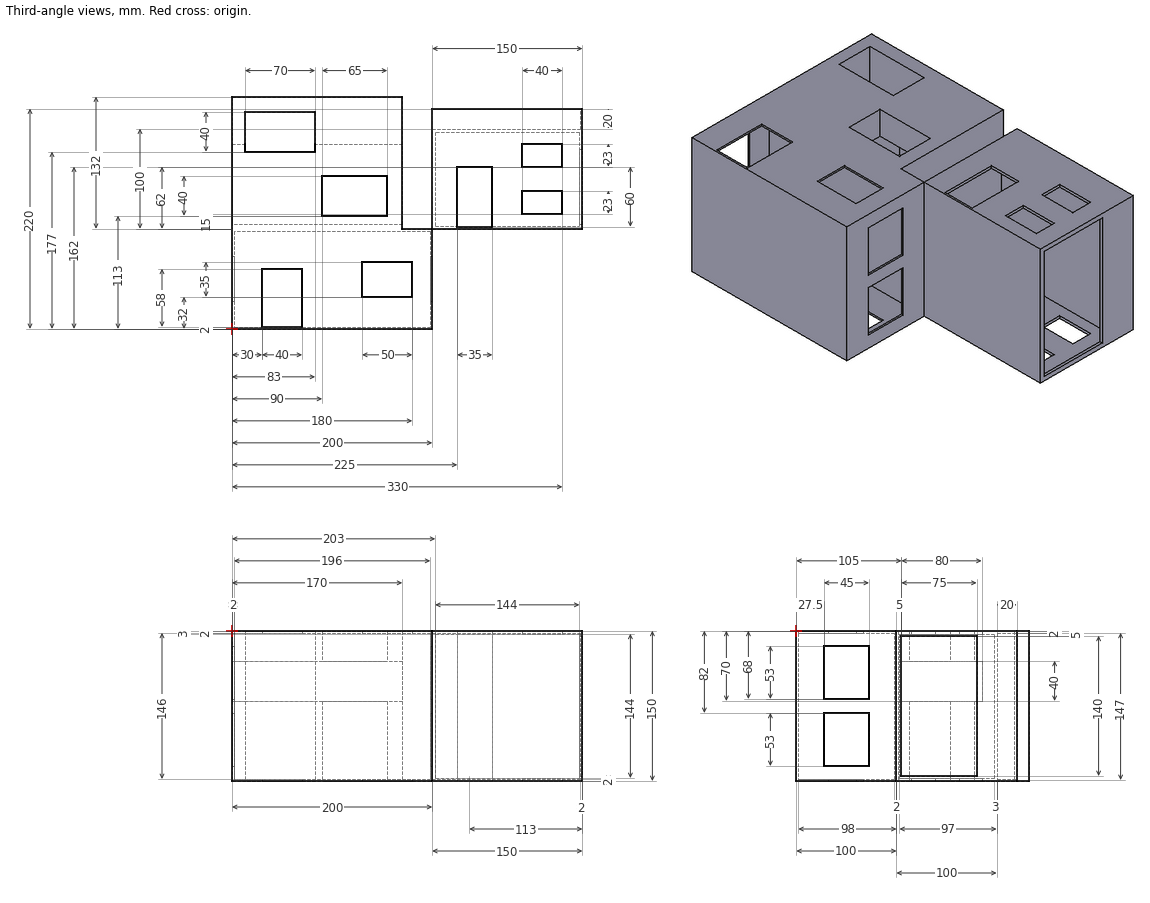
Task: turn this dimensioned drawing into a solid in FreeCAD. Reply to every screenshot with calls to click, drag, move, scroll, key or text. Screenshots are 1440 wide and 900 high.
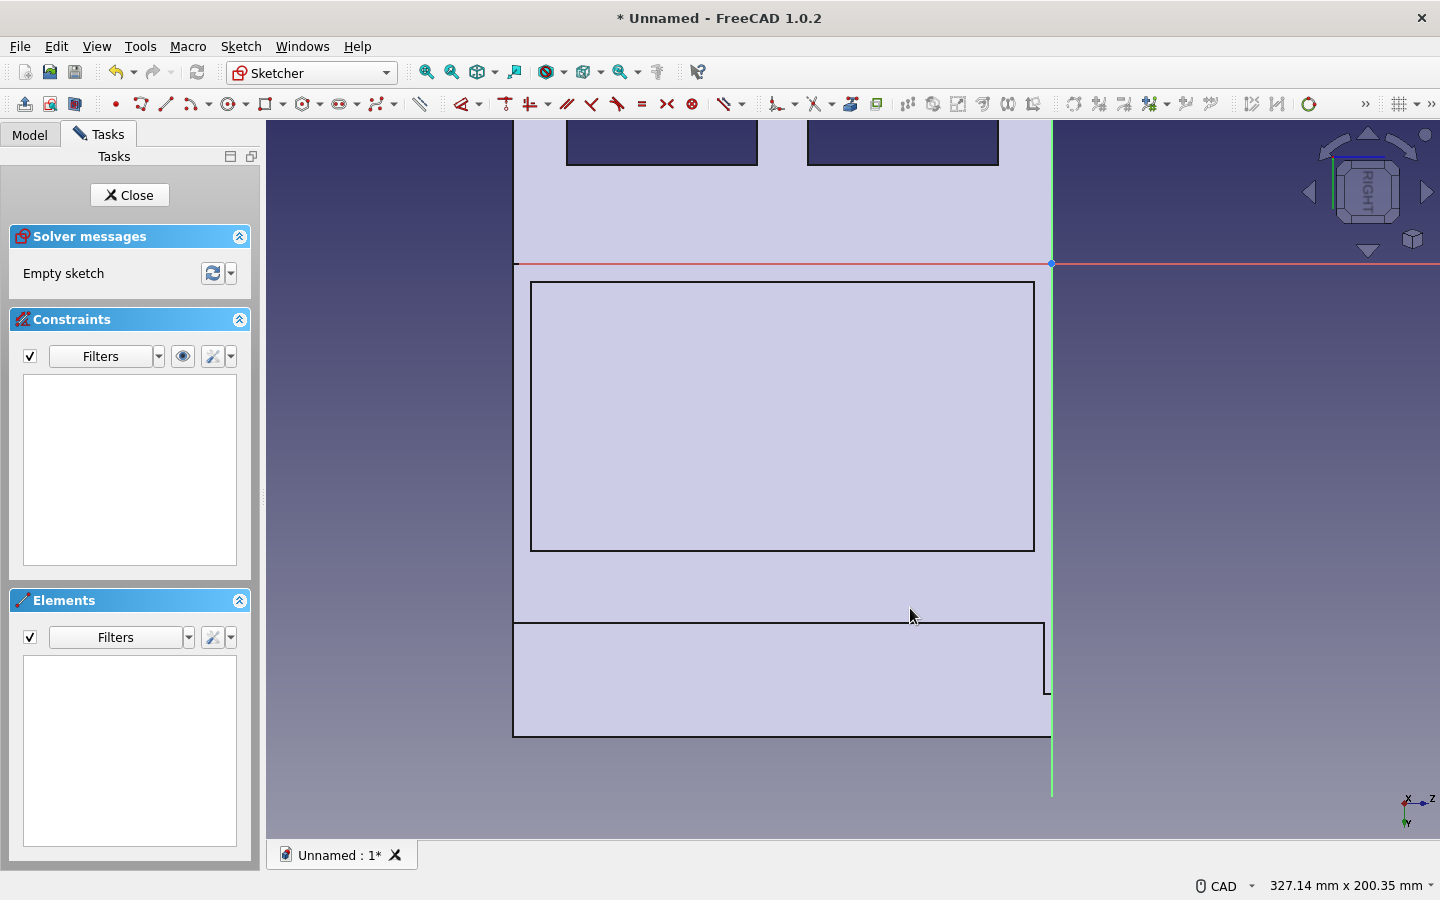
click(264, 104)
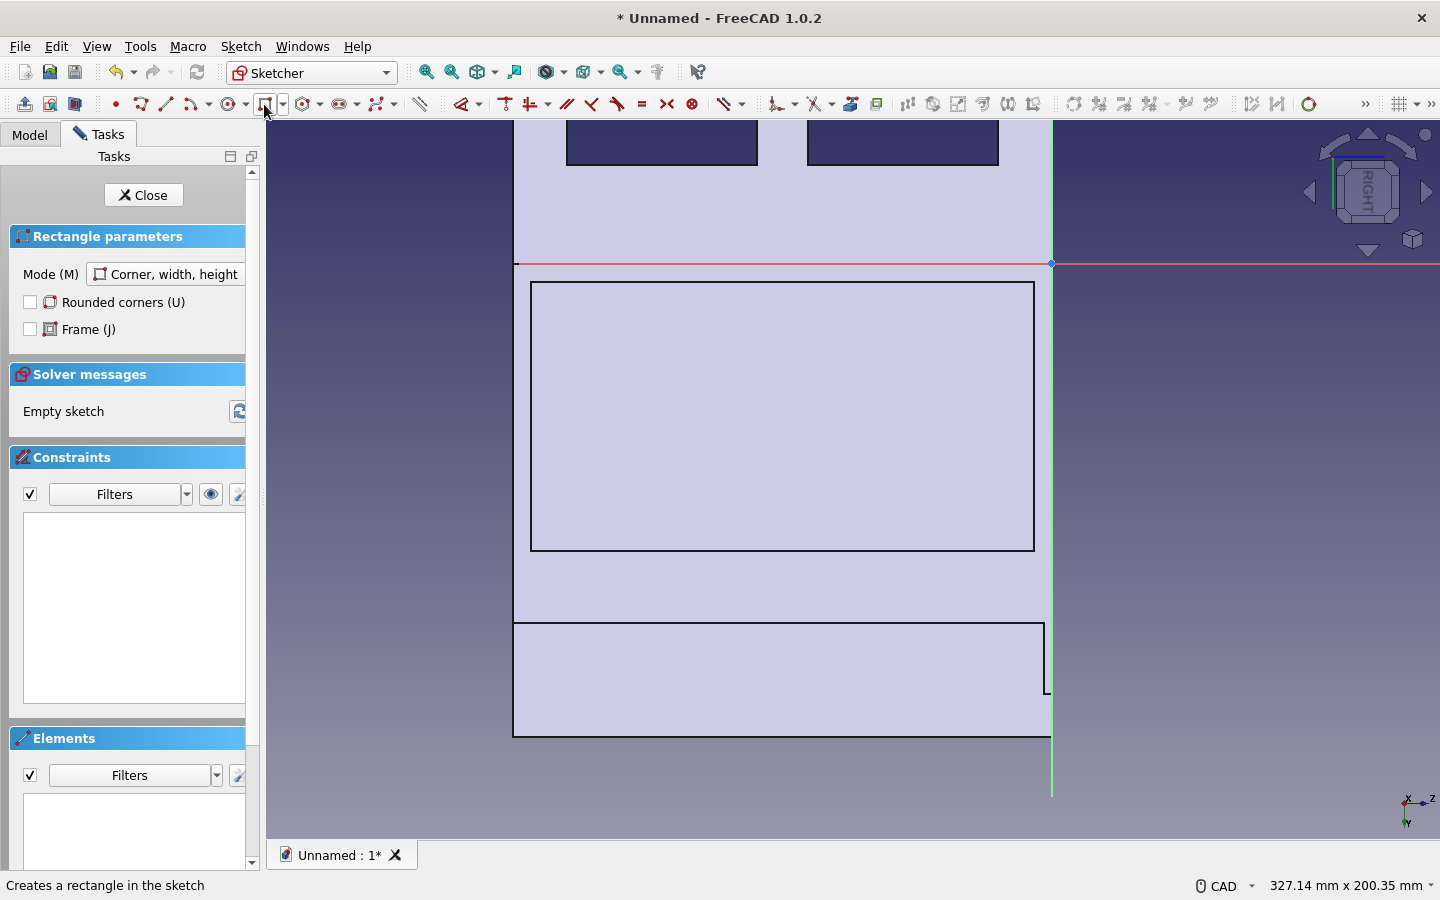
click(517, 623)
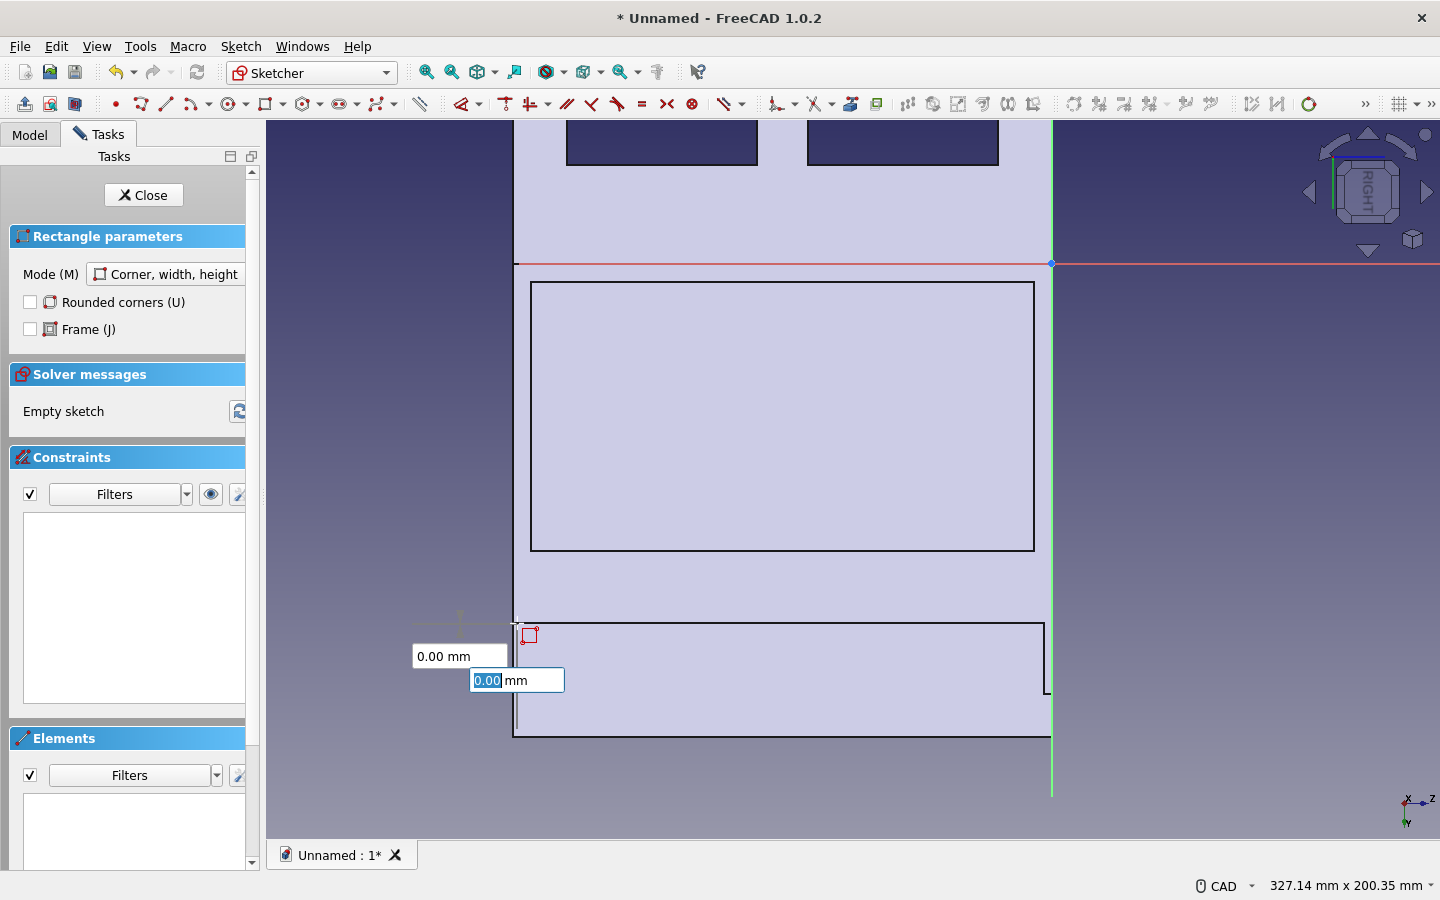
scroll(1044, 694, up, 4)
move(1044, 694)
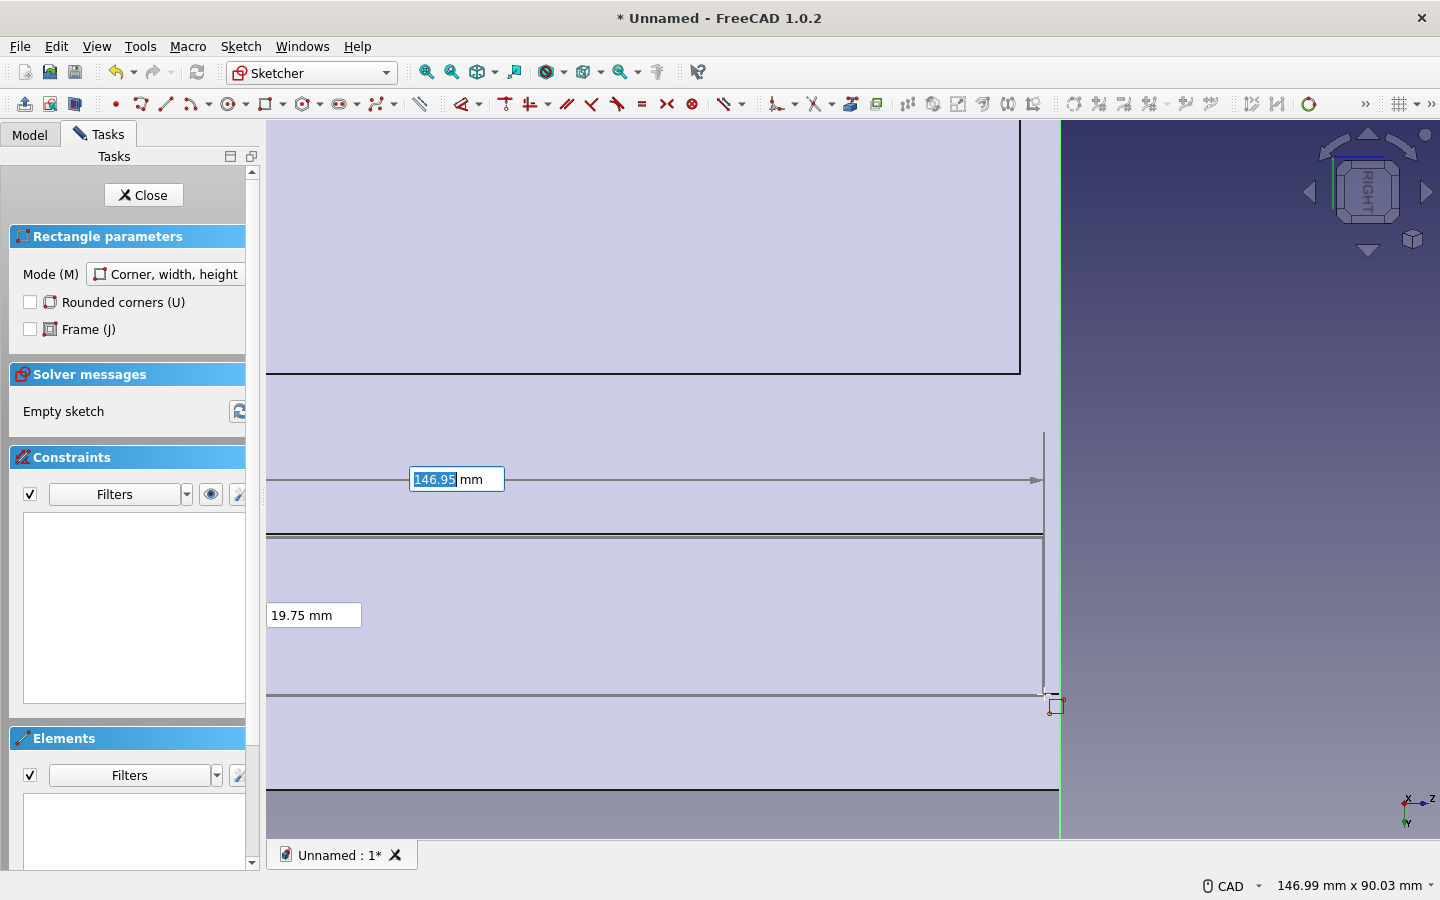
text(147)
key(Tab)
text(20)
key(Return)
key(Escape)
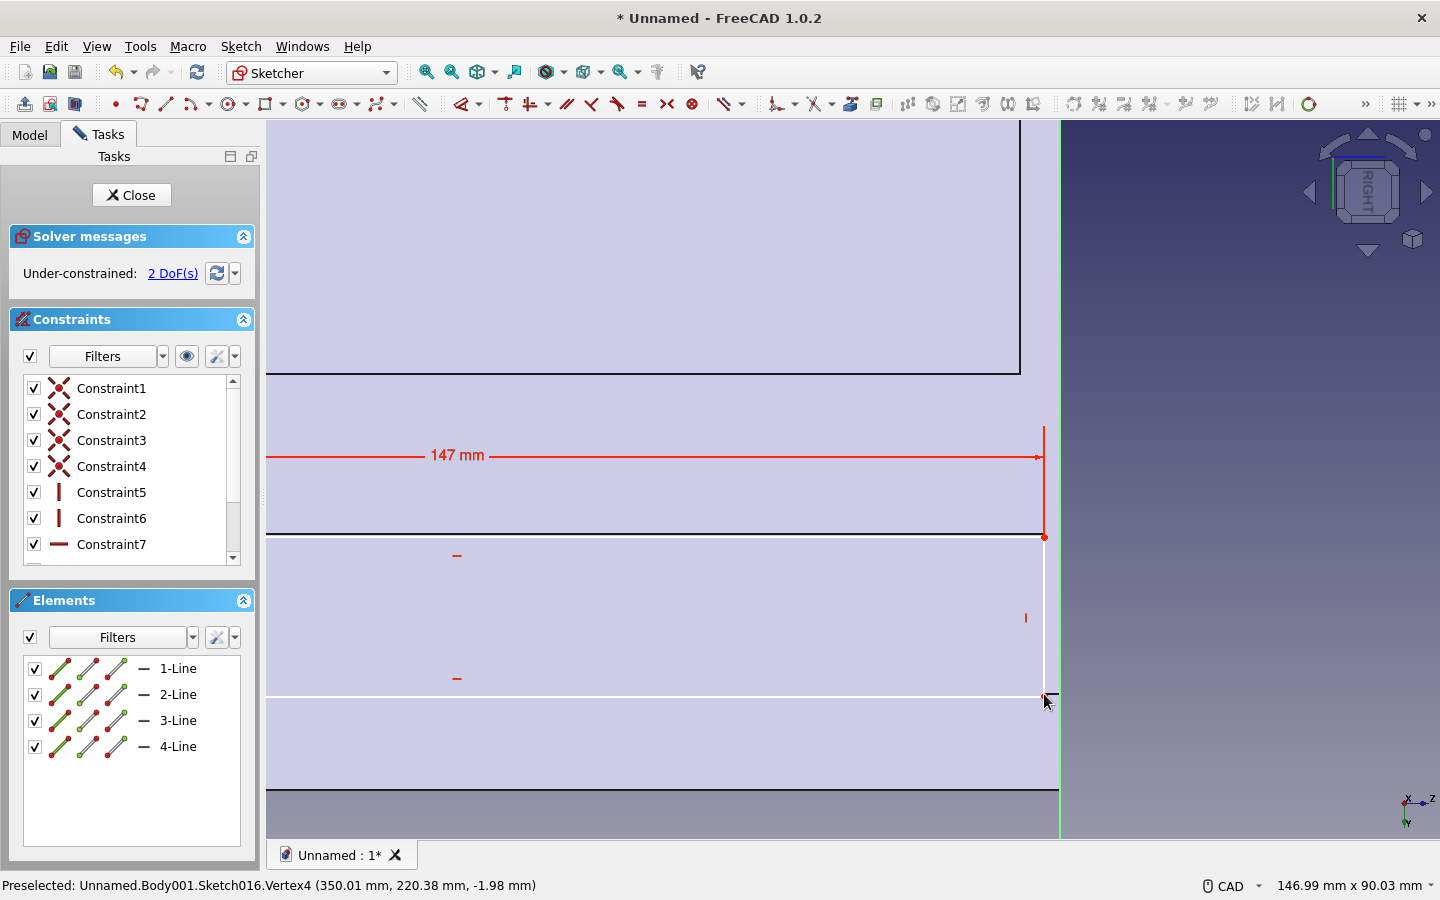
click(460, 104)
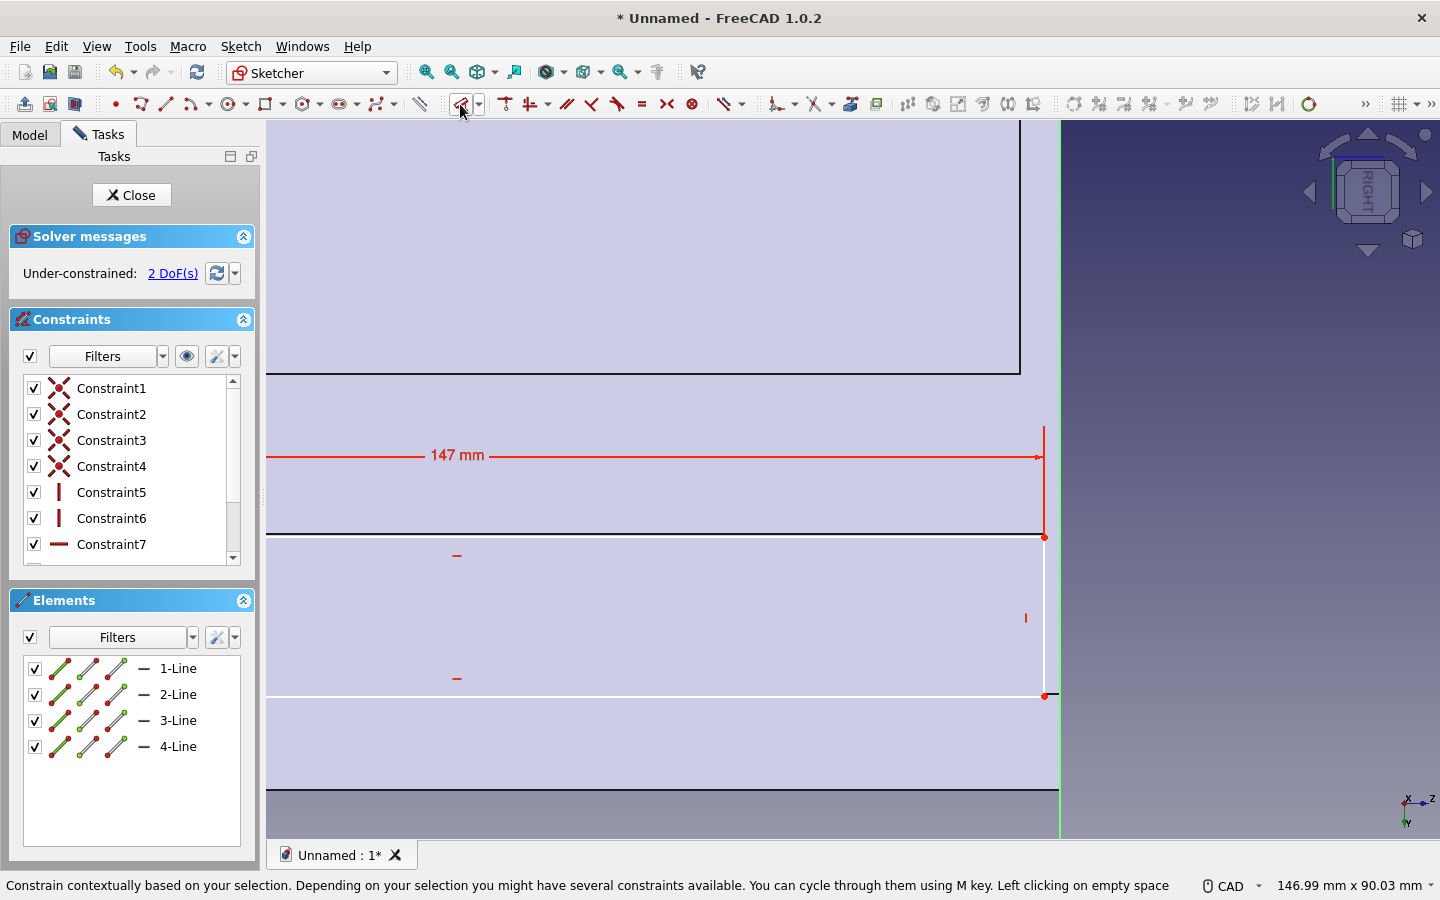
scroll(1044, 697, up, 5)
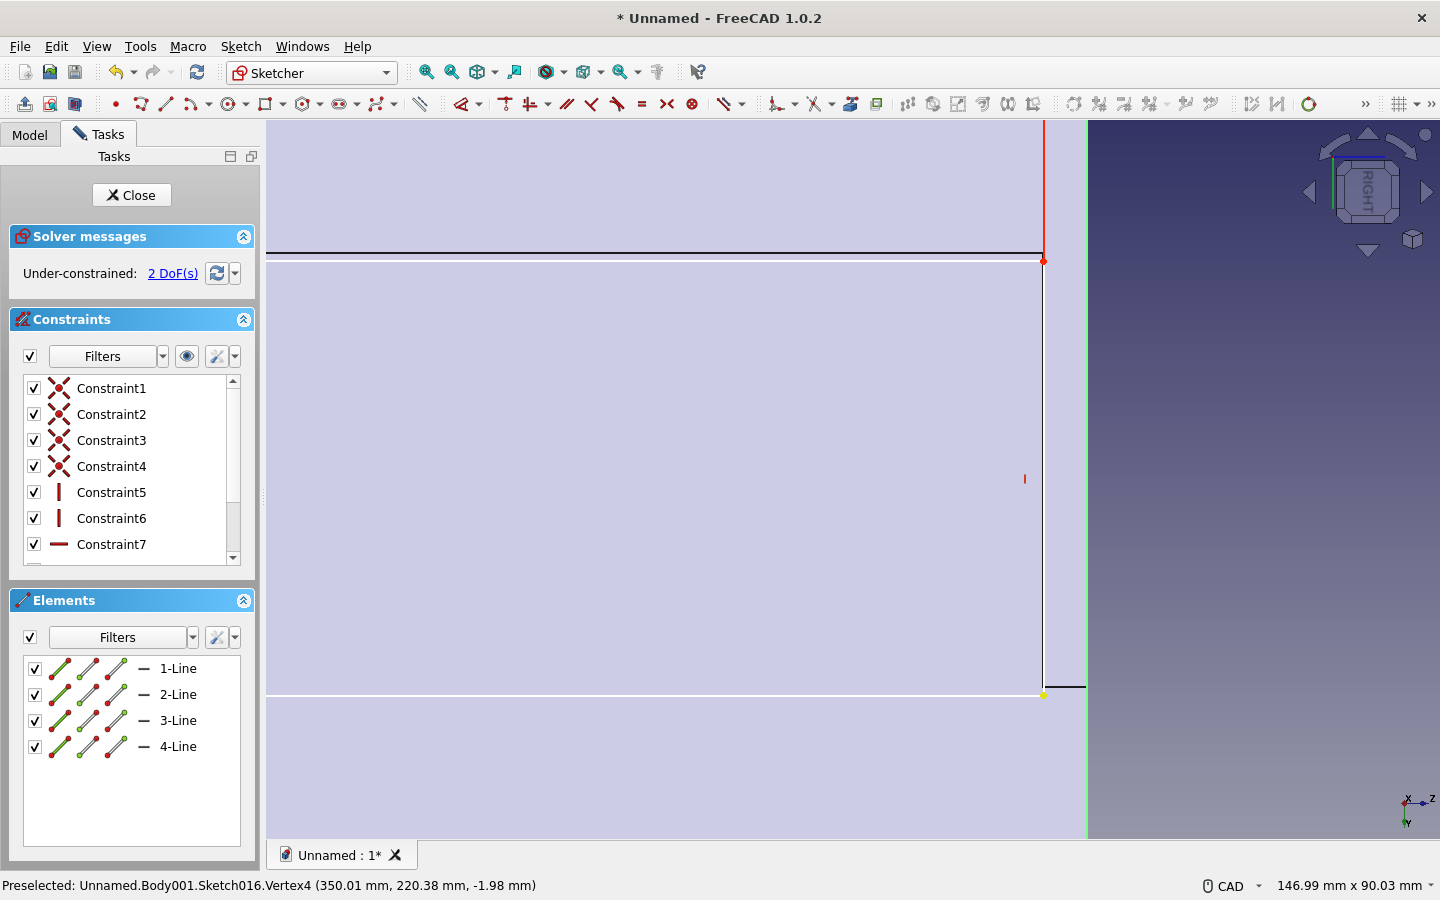
click(1044, 696)
click(1065, 730)